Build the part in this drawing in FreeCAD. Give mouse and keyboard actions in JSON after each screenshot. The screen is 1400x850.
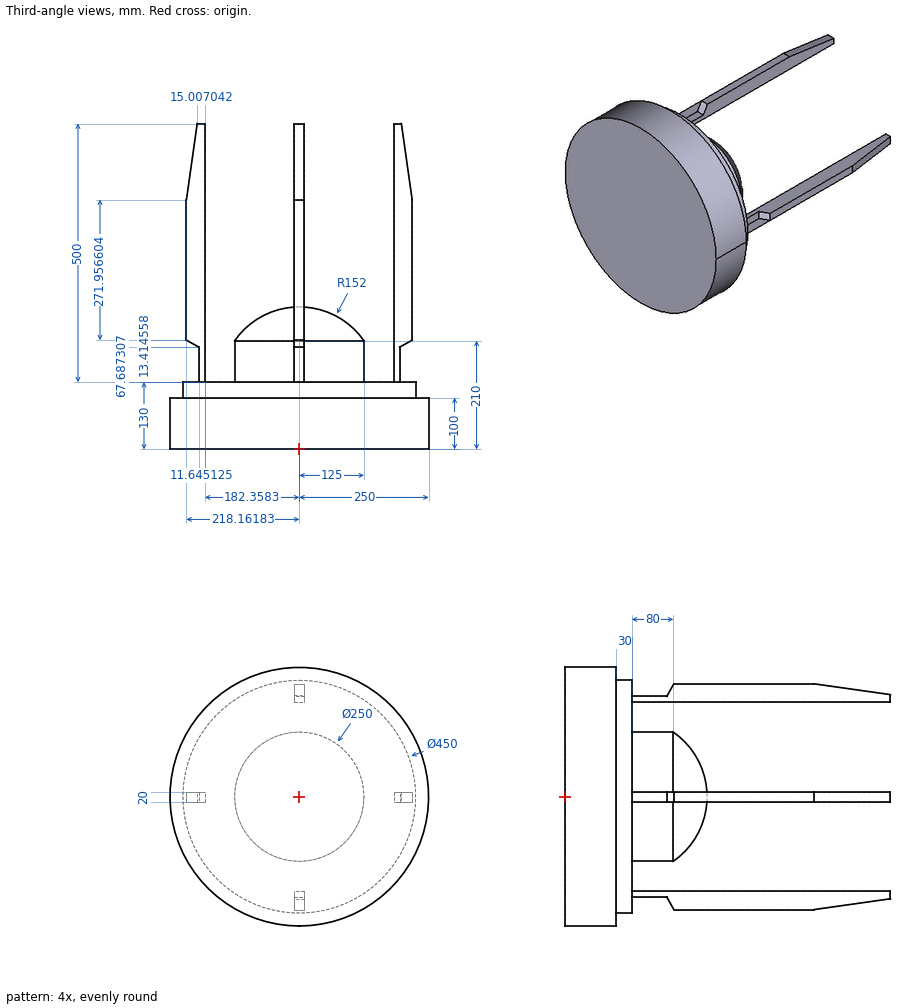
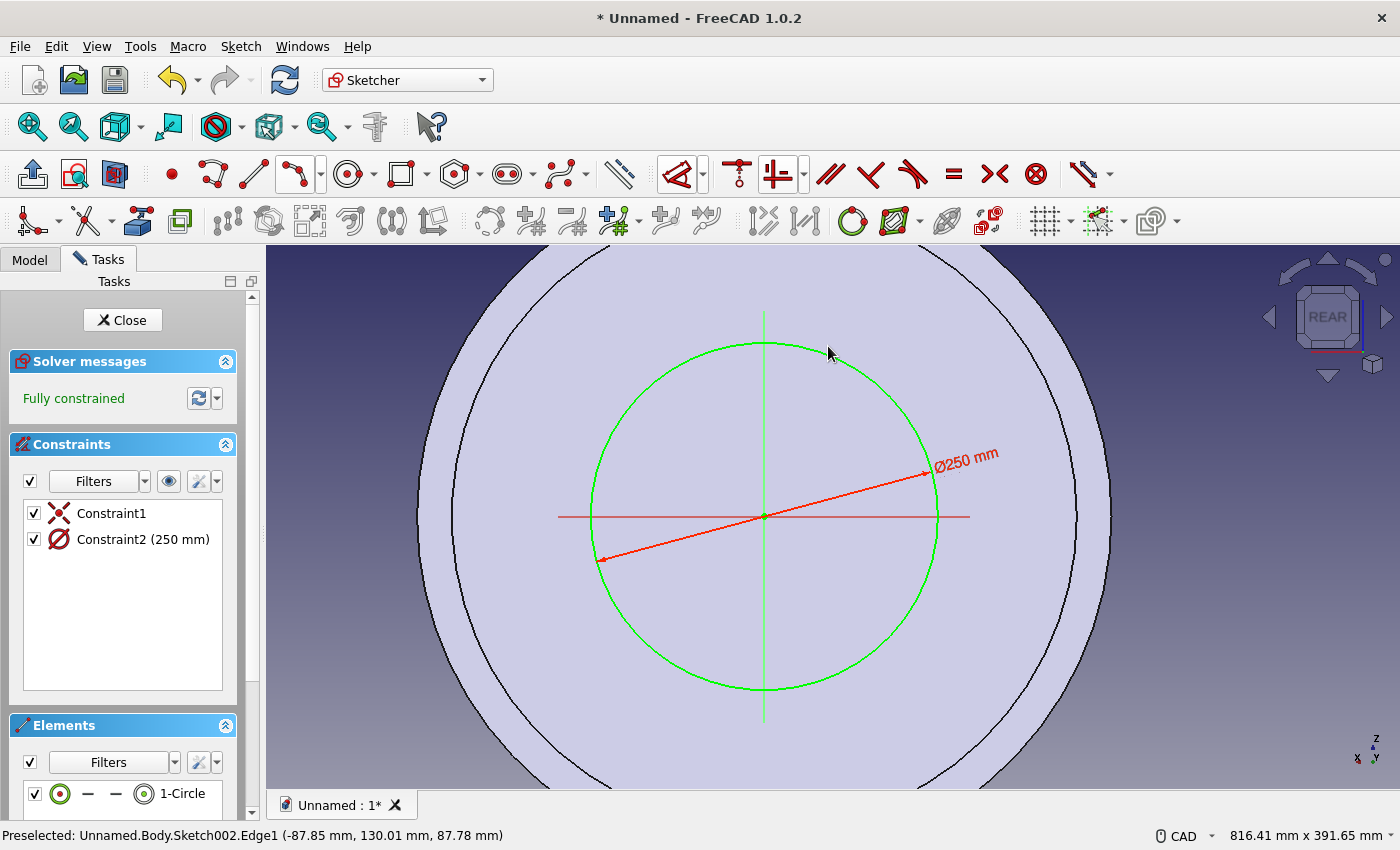
{"action": "left_click", "coordinate": [123, 320]}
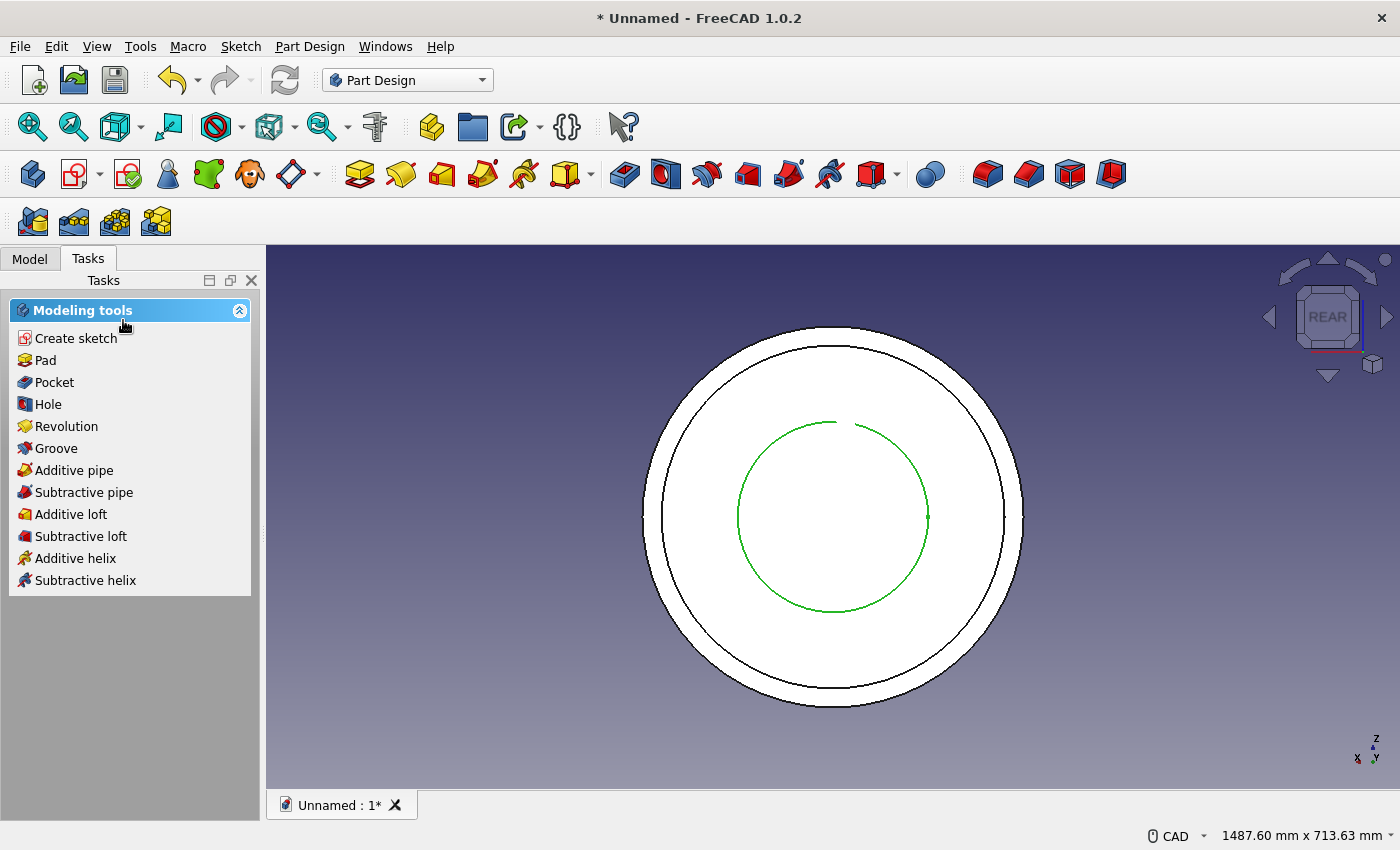
{"action": "left_click", "coordinate": [360, 174]}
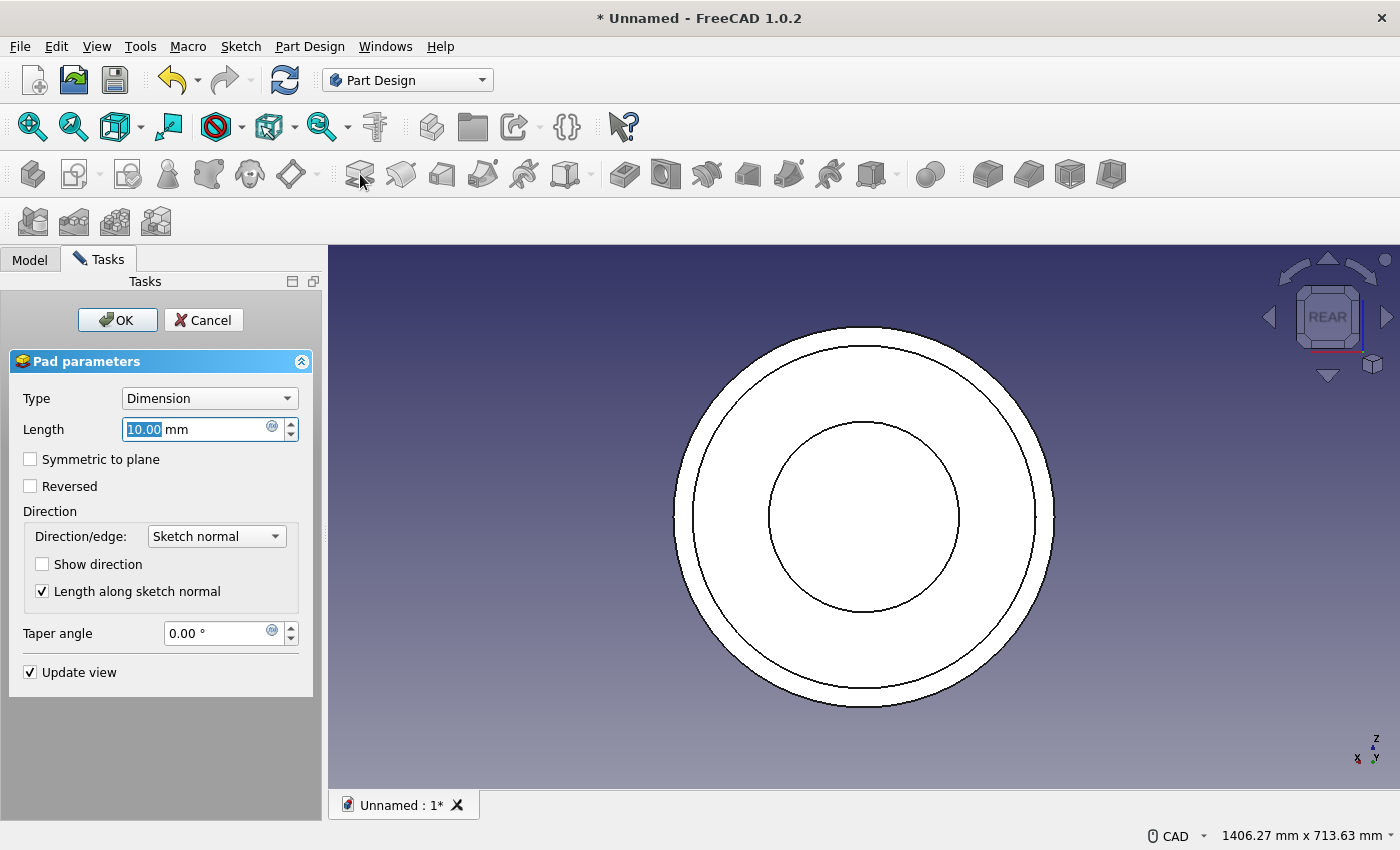
{"action": "type", "text": "80"}
{"action": "key", "text": "Tab"}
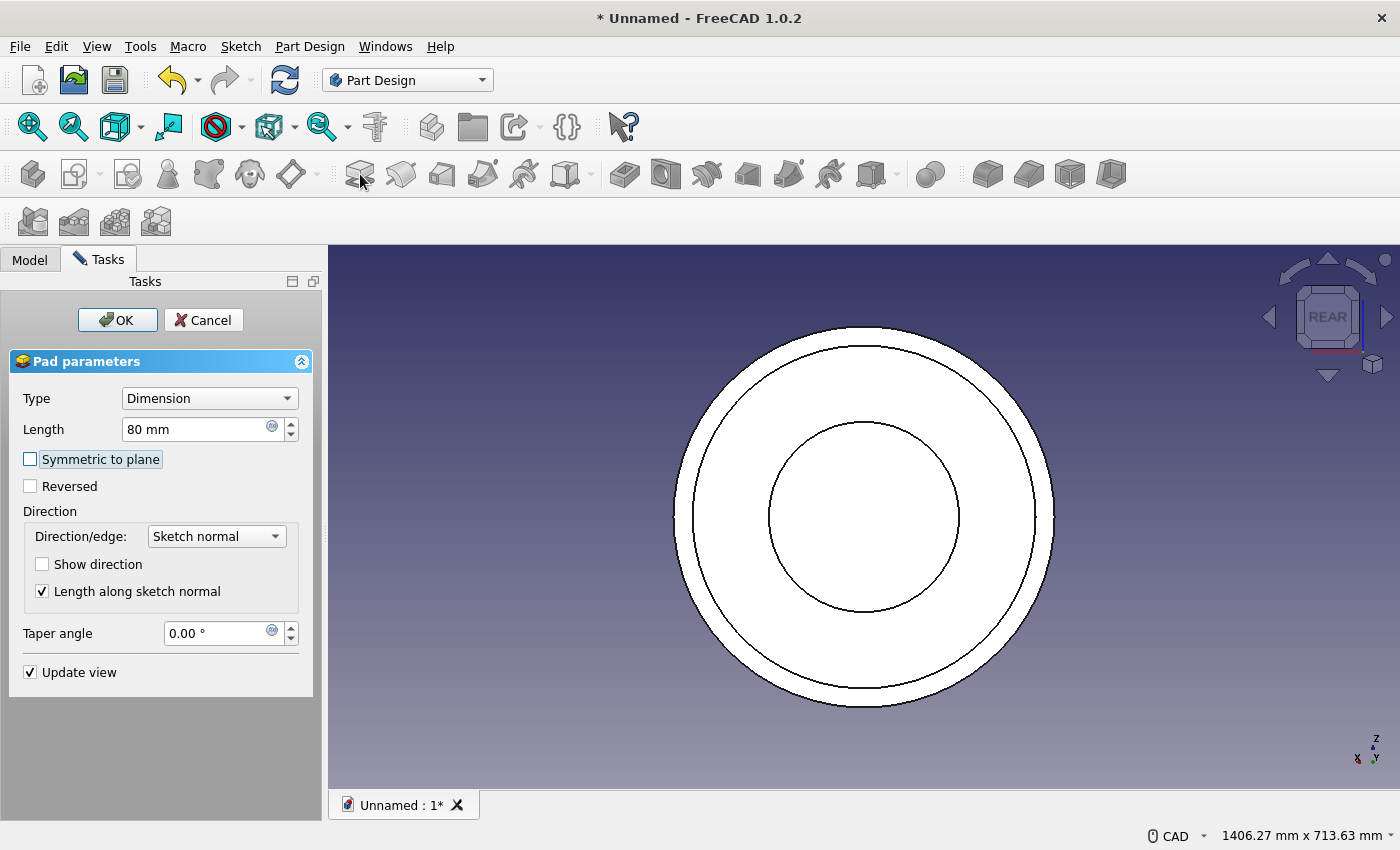
{"action": "left_click", "coordinate": [118, 320]}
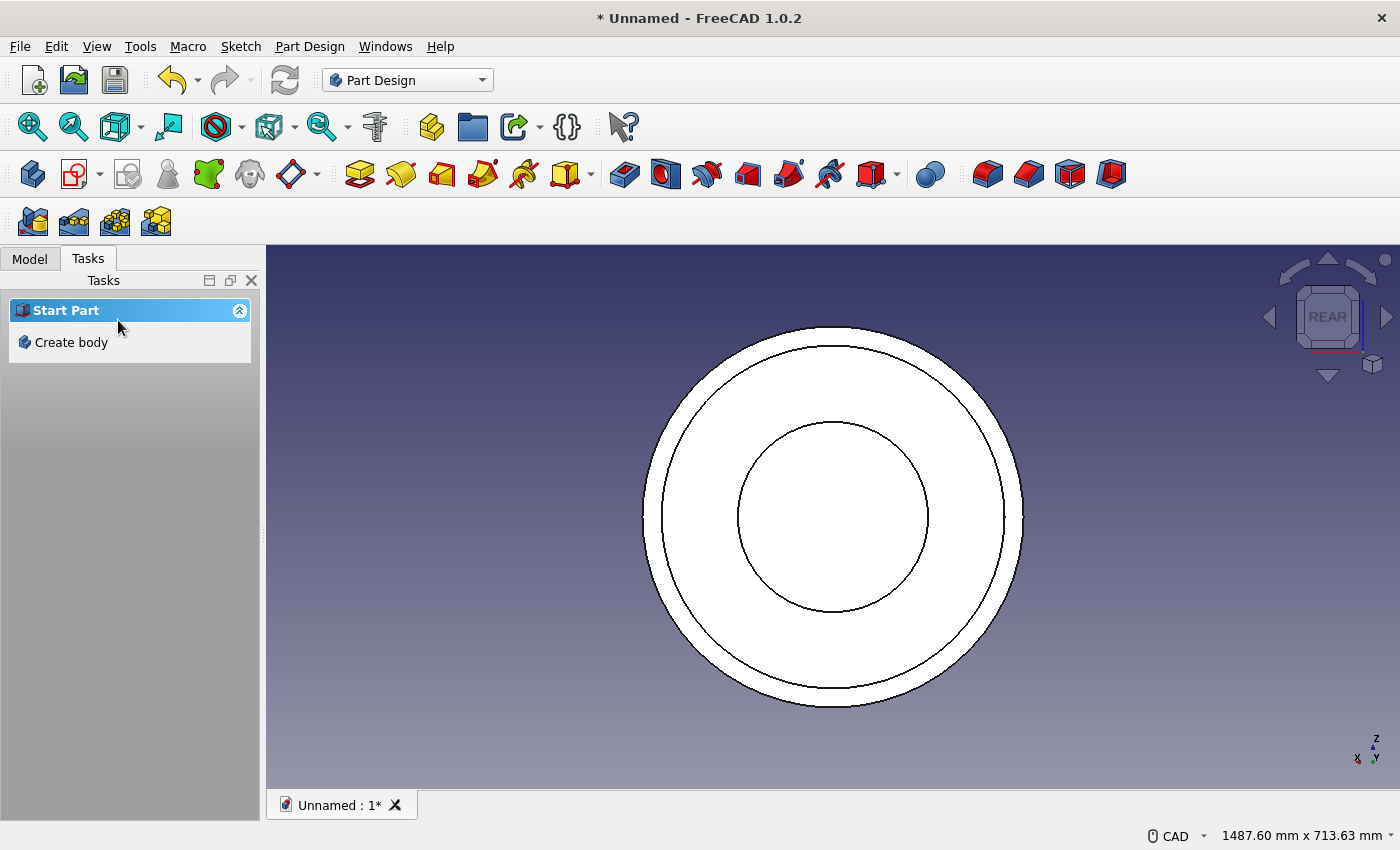
{"action": "left_click", "coordinate": [74, 174]}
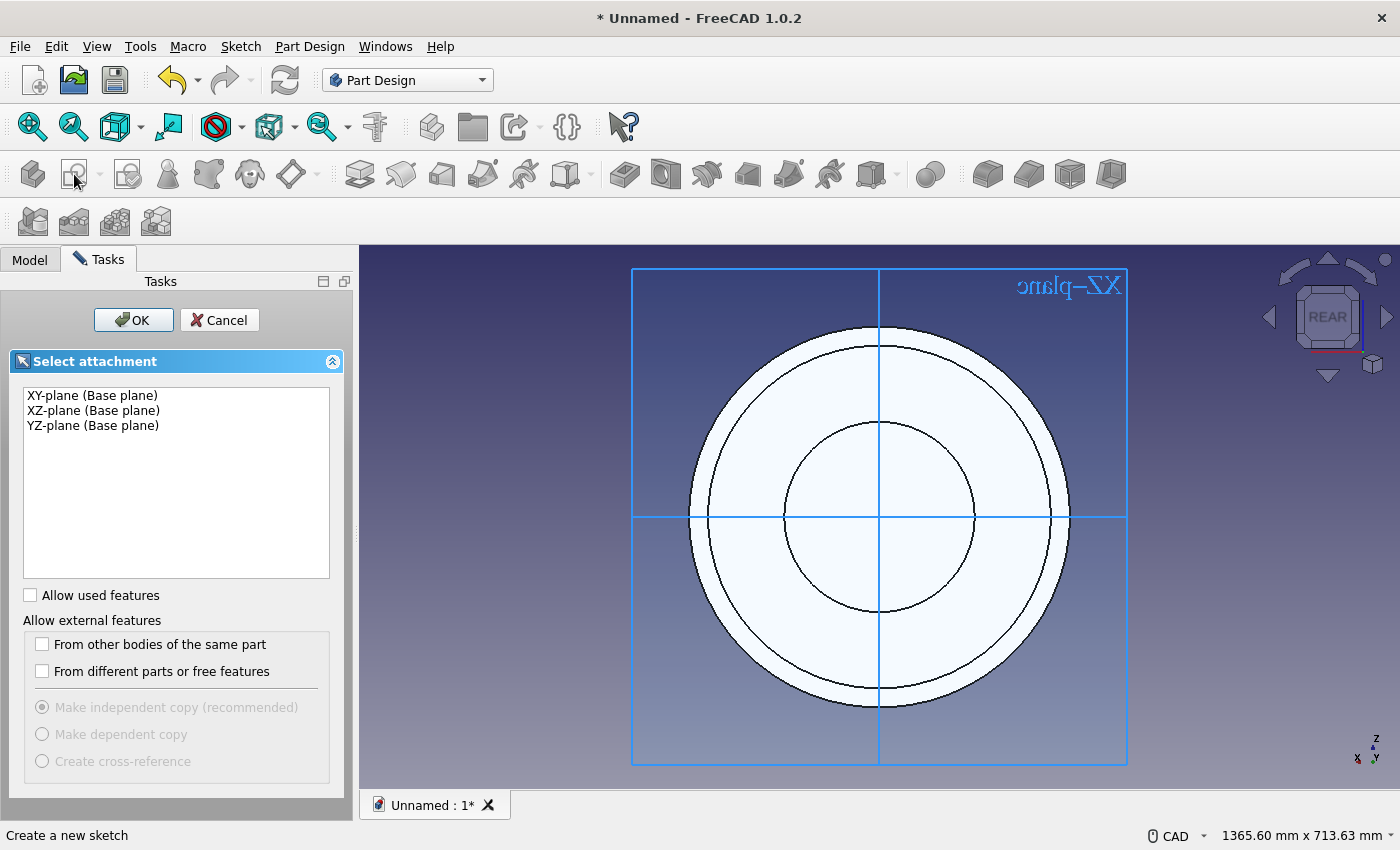
{"action": "left_click", "coordinate": [84, 396]}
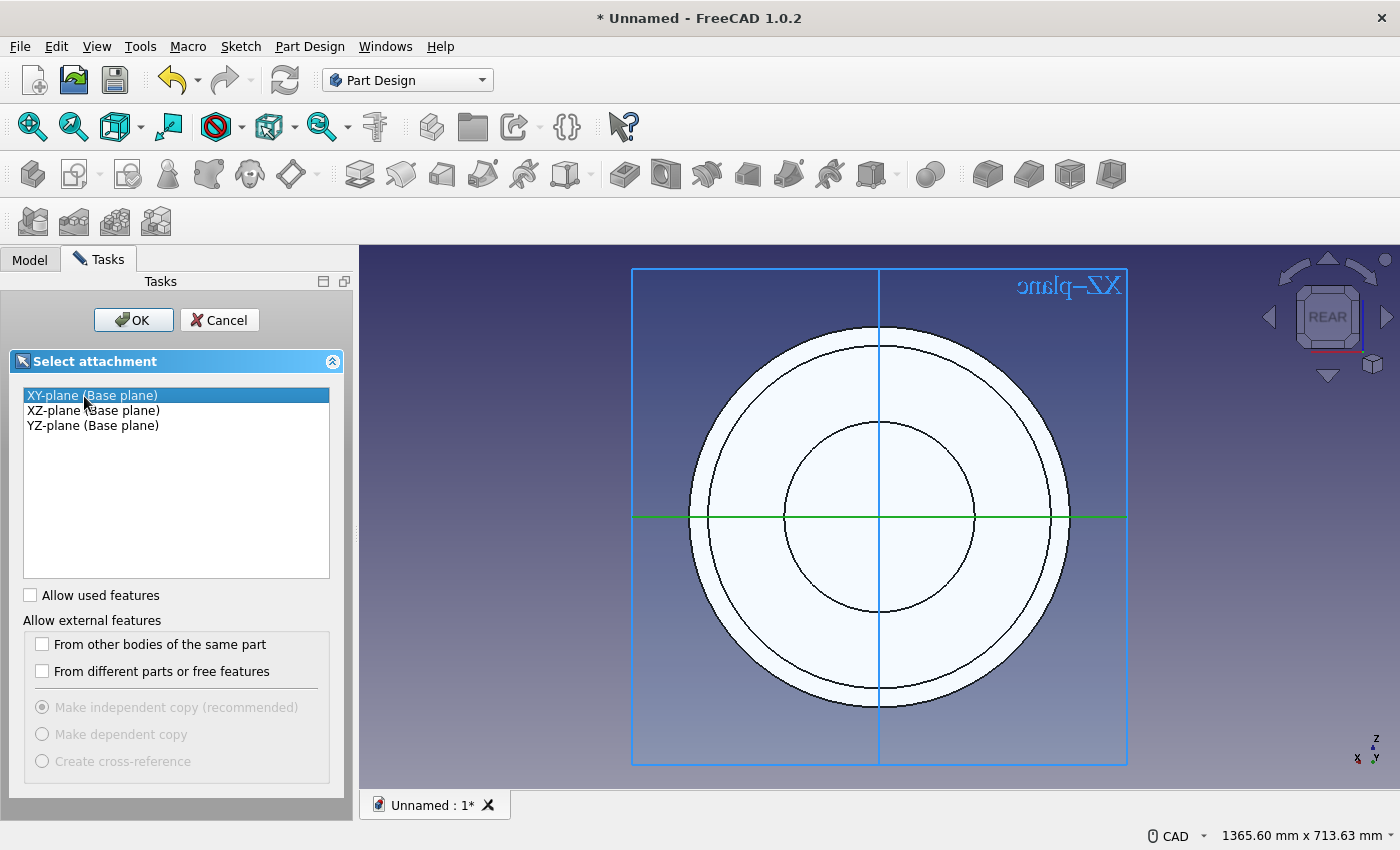
{"action": "left_click", "coordinate": [134, 320]}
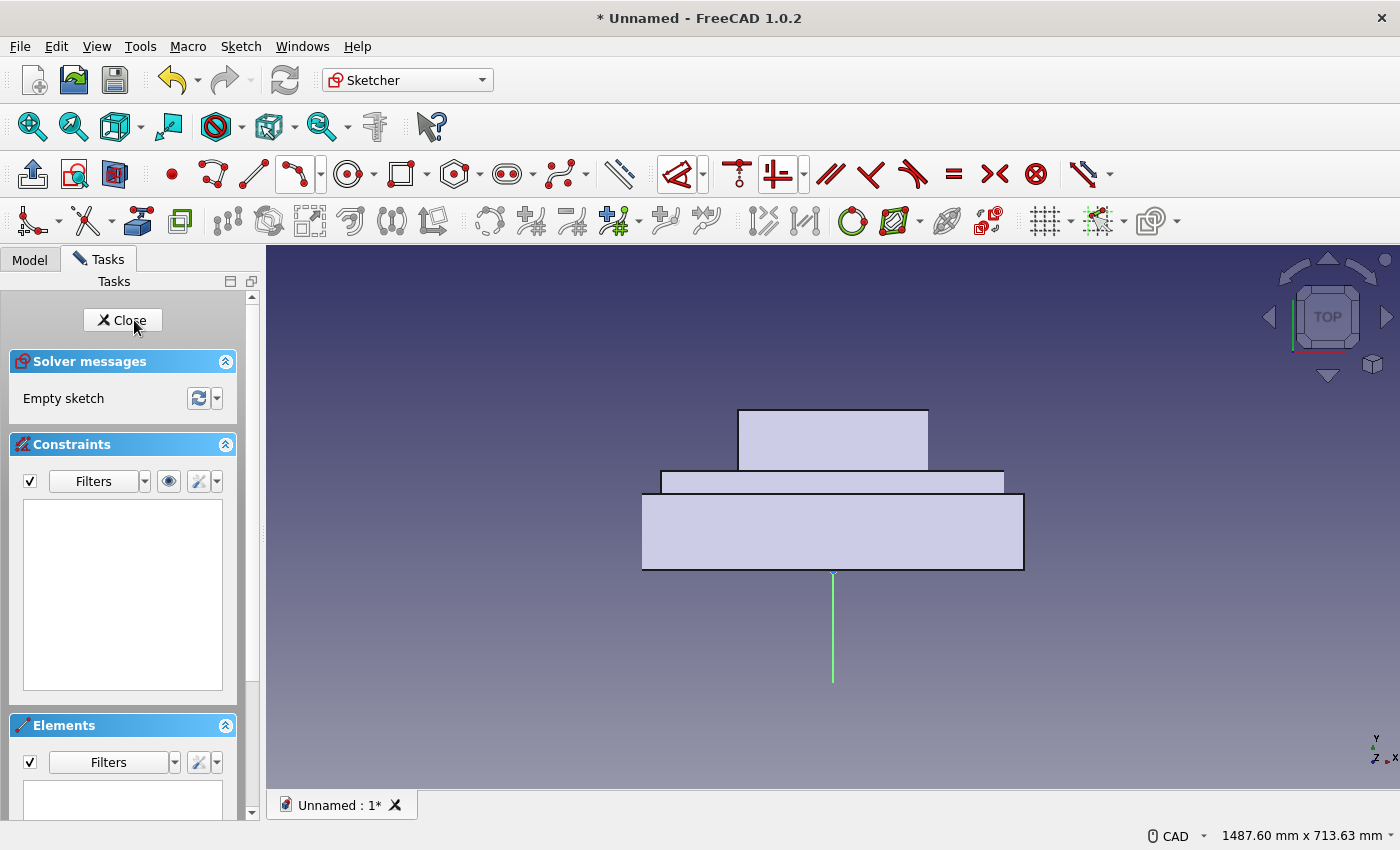
{"action": "left_click", "coordinate": [115, 174]}